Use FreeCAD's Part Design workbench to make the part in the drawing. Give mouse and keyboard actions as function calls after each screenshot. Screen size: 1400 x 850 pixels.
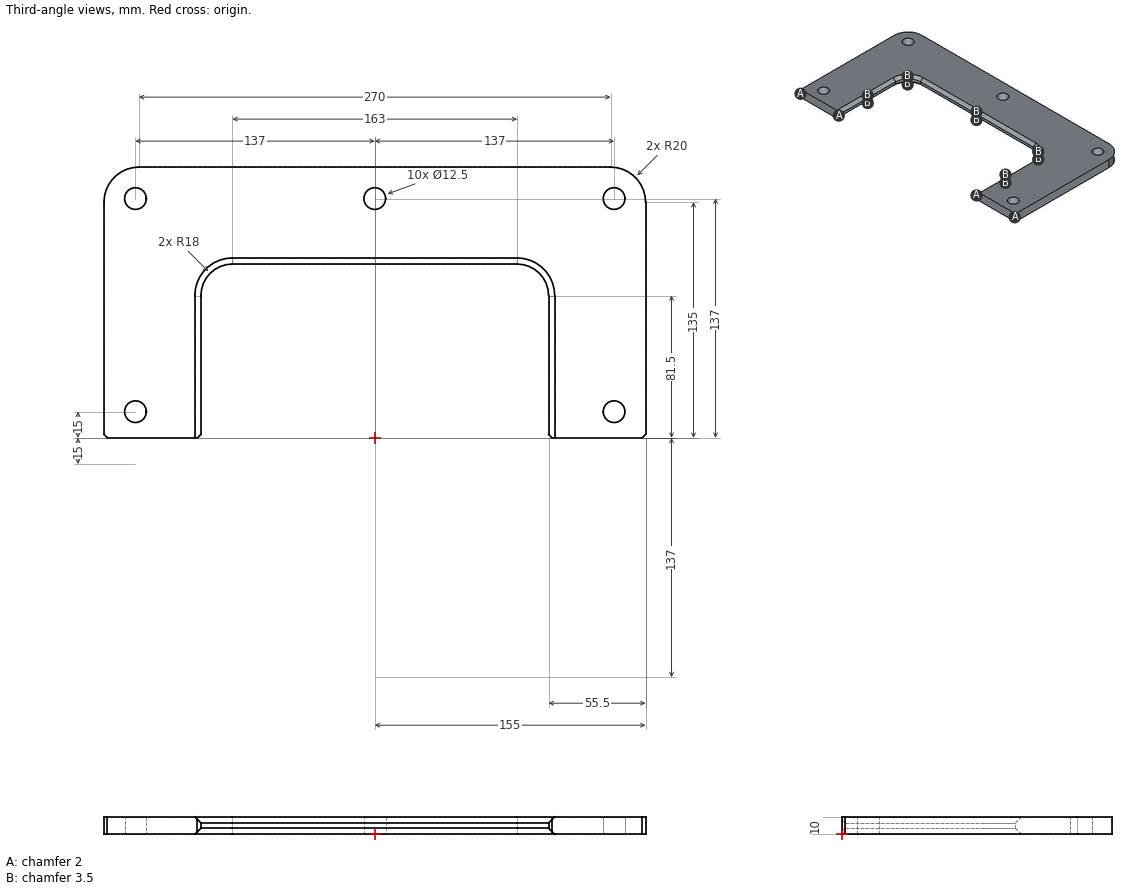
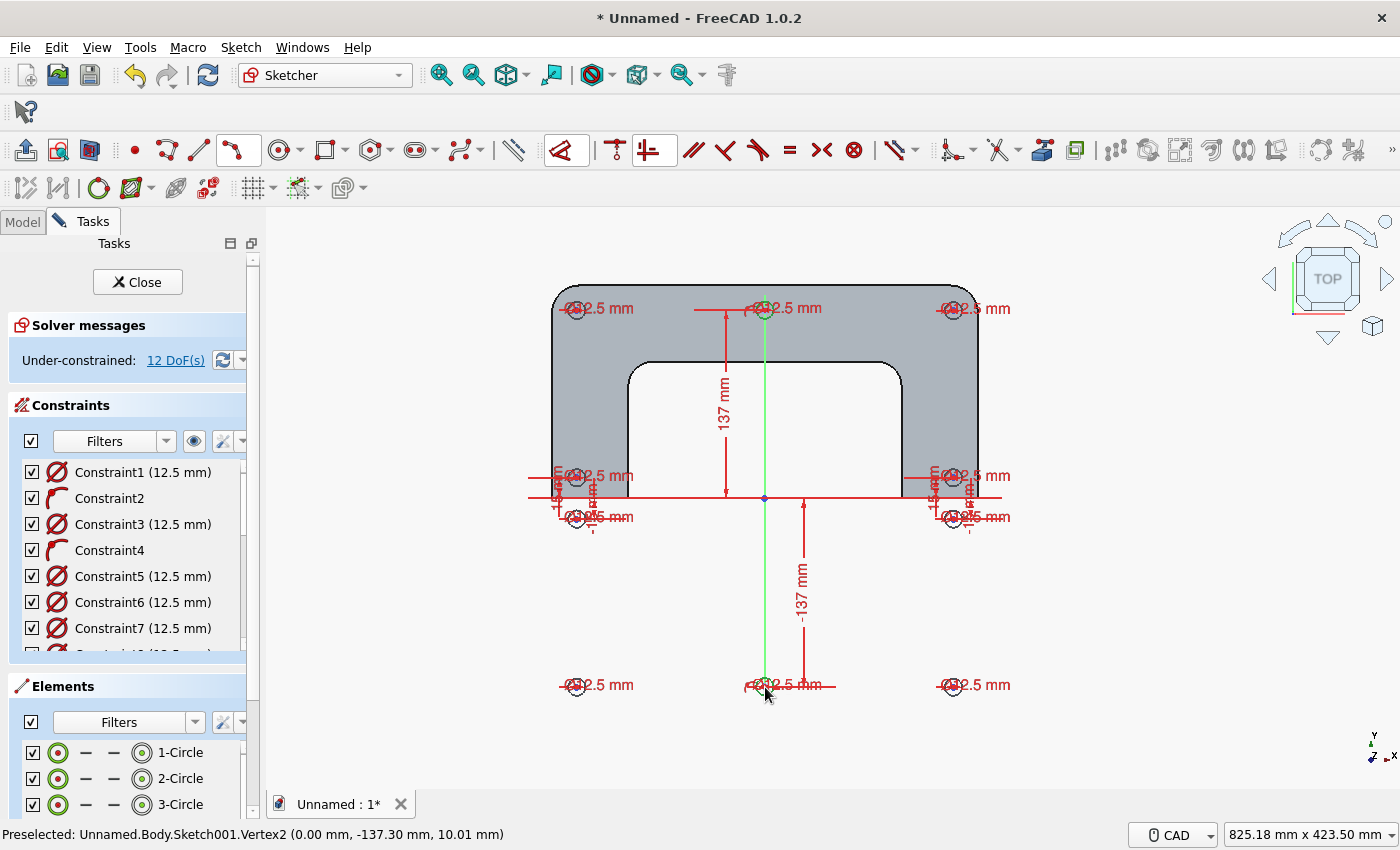
click(577, 310)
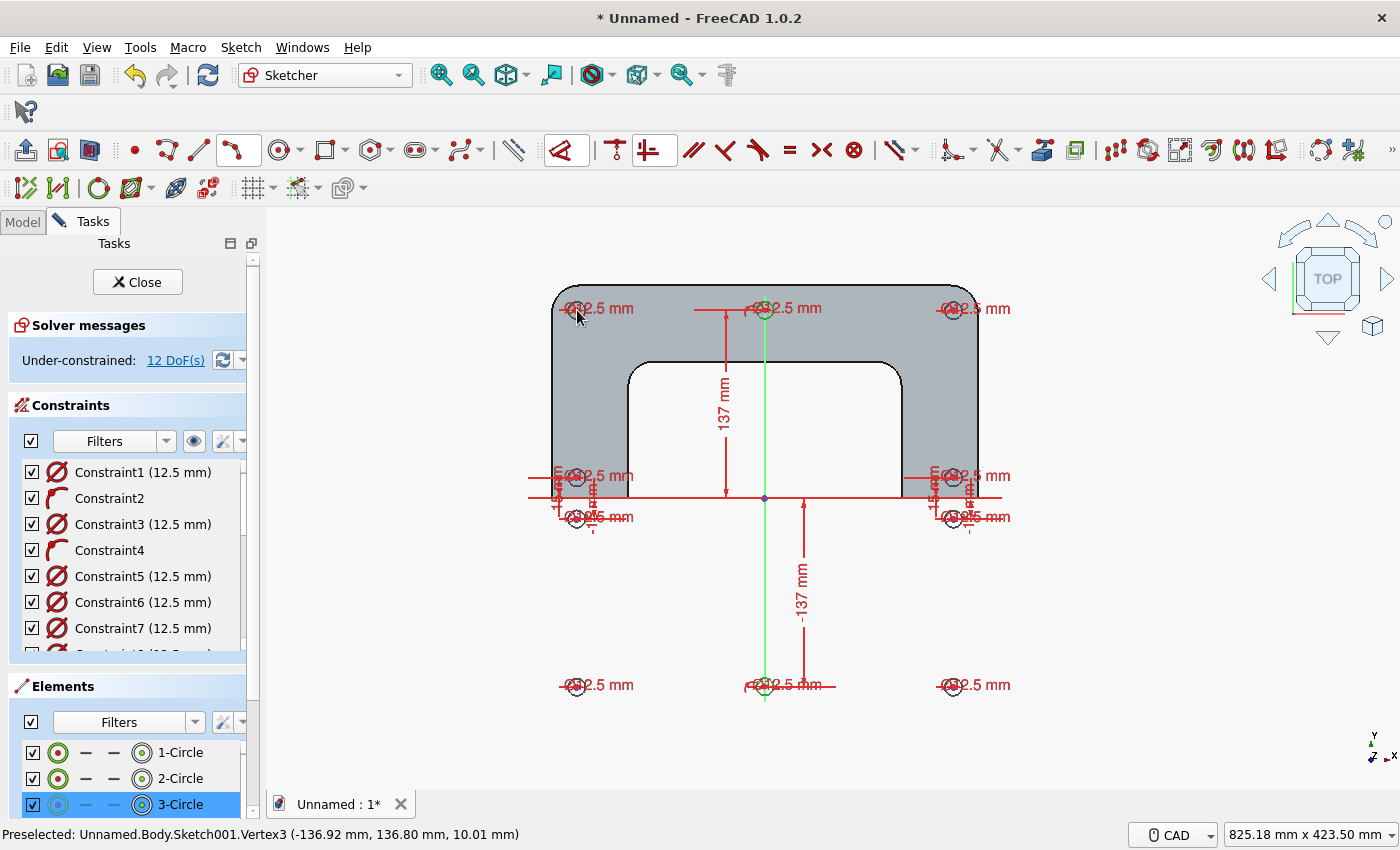
key(l)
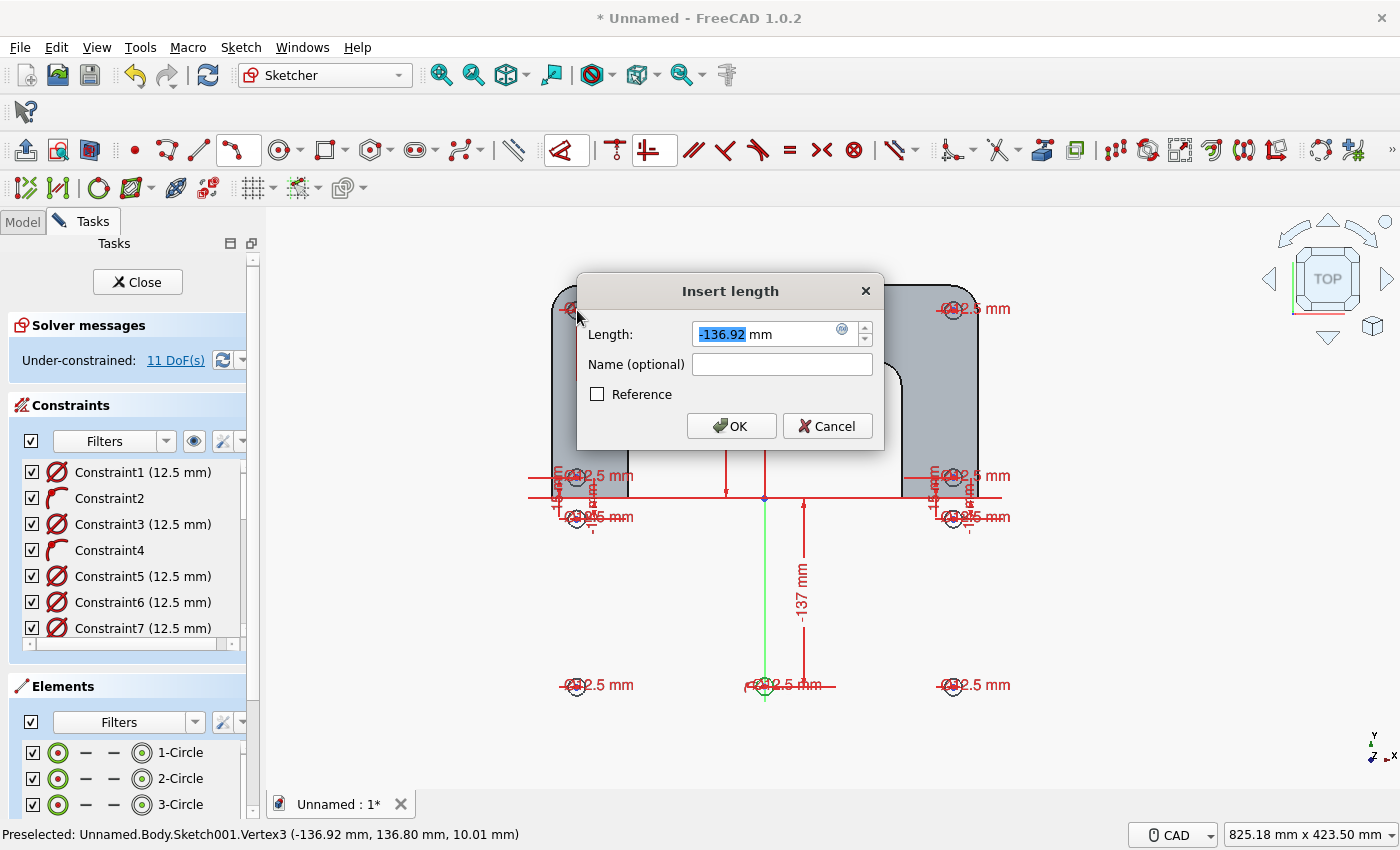
text(-137)
key(Return)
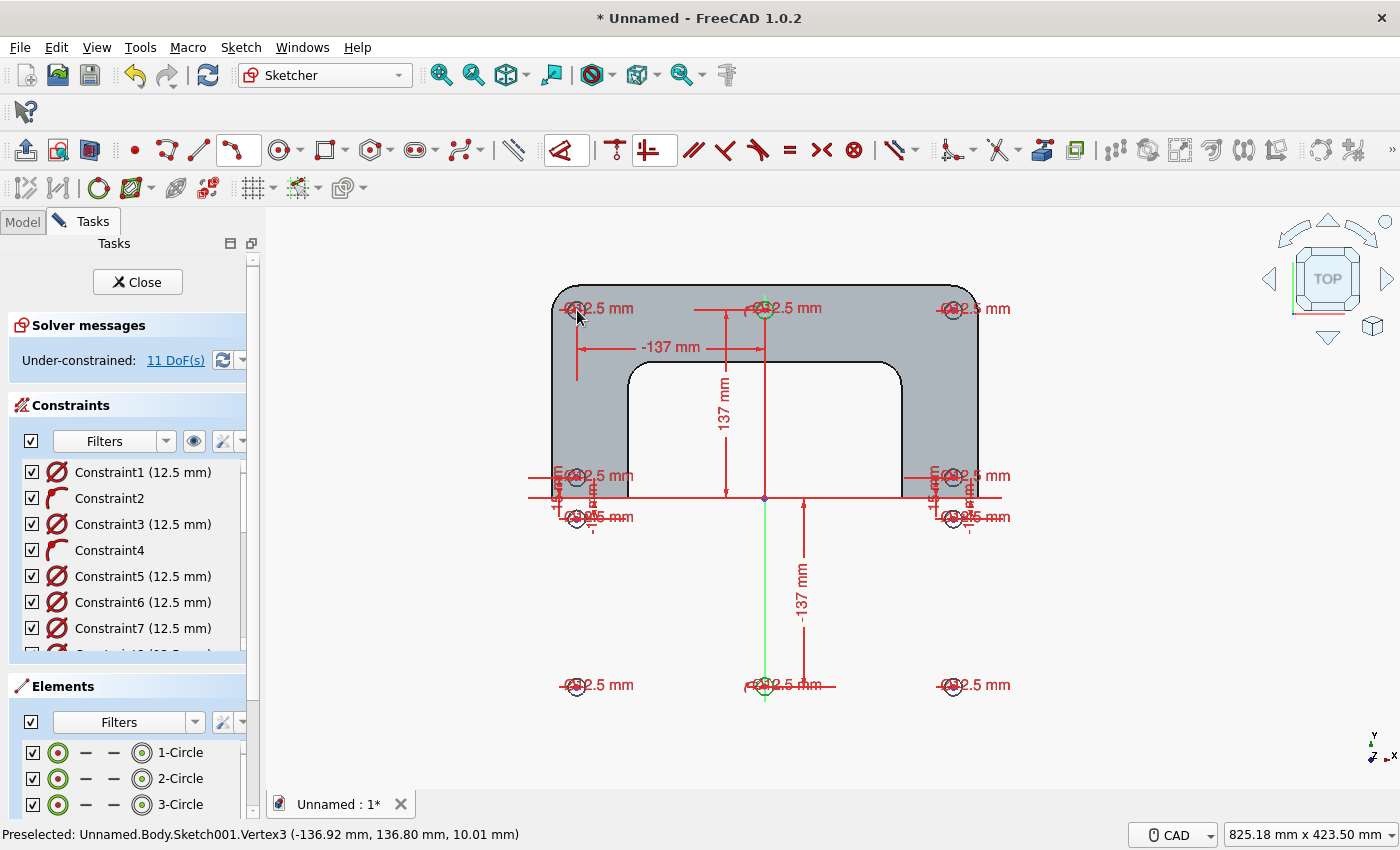
click(577, 310)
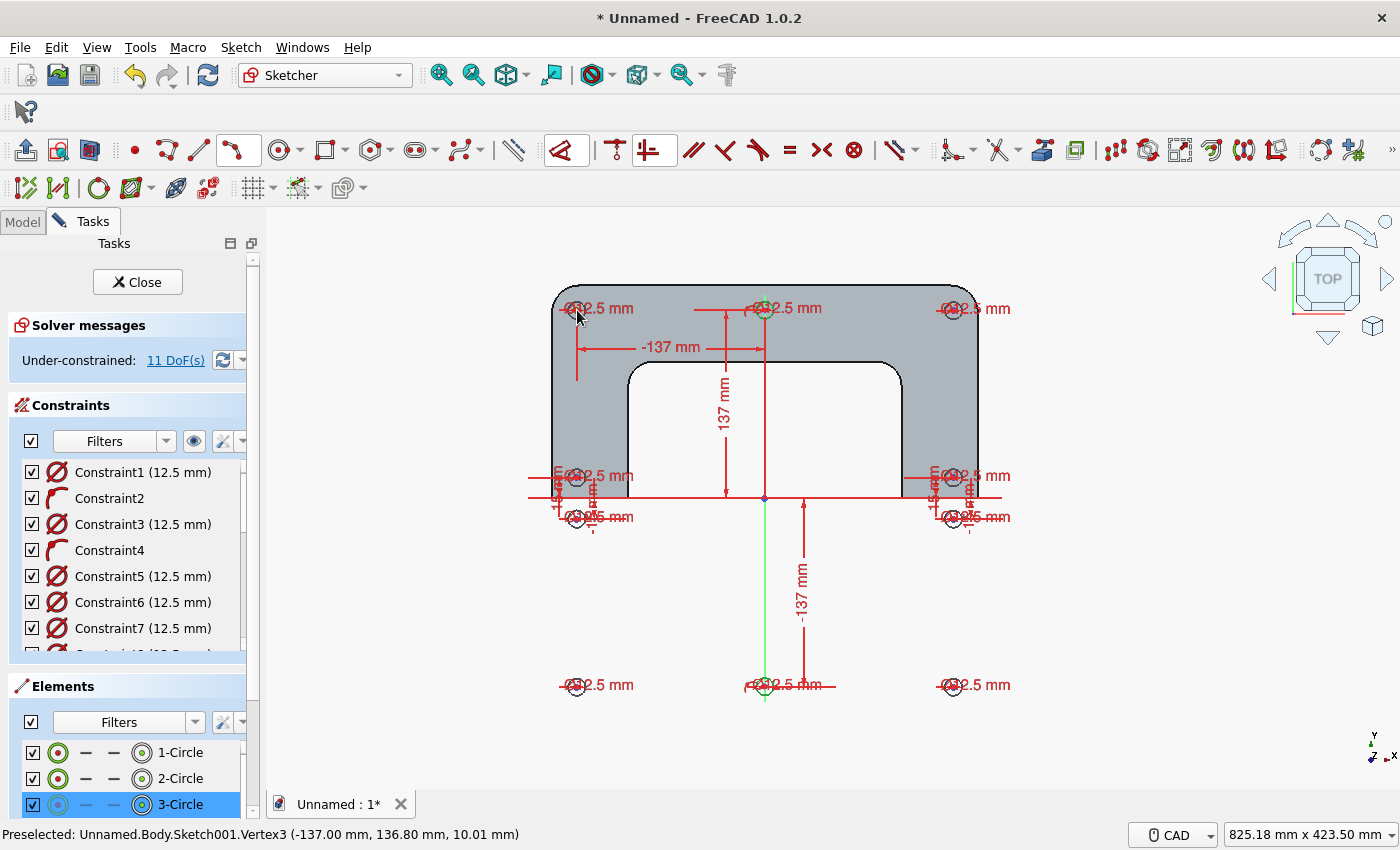
key(i)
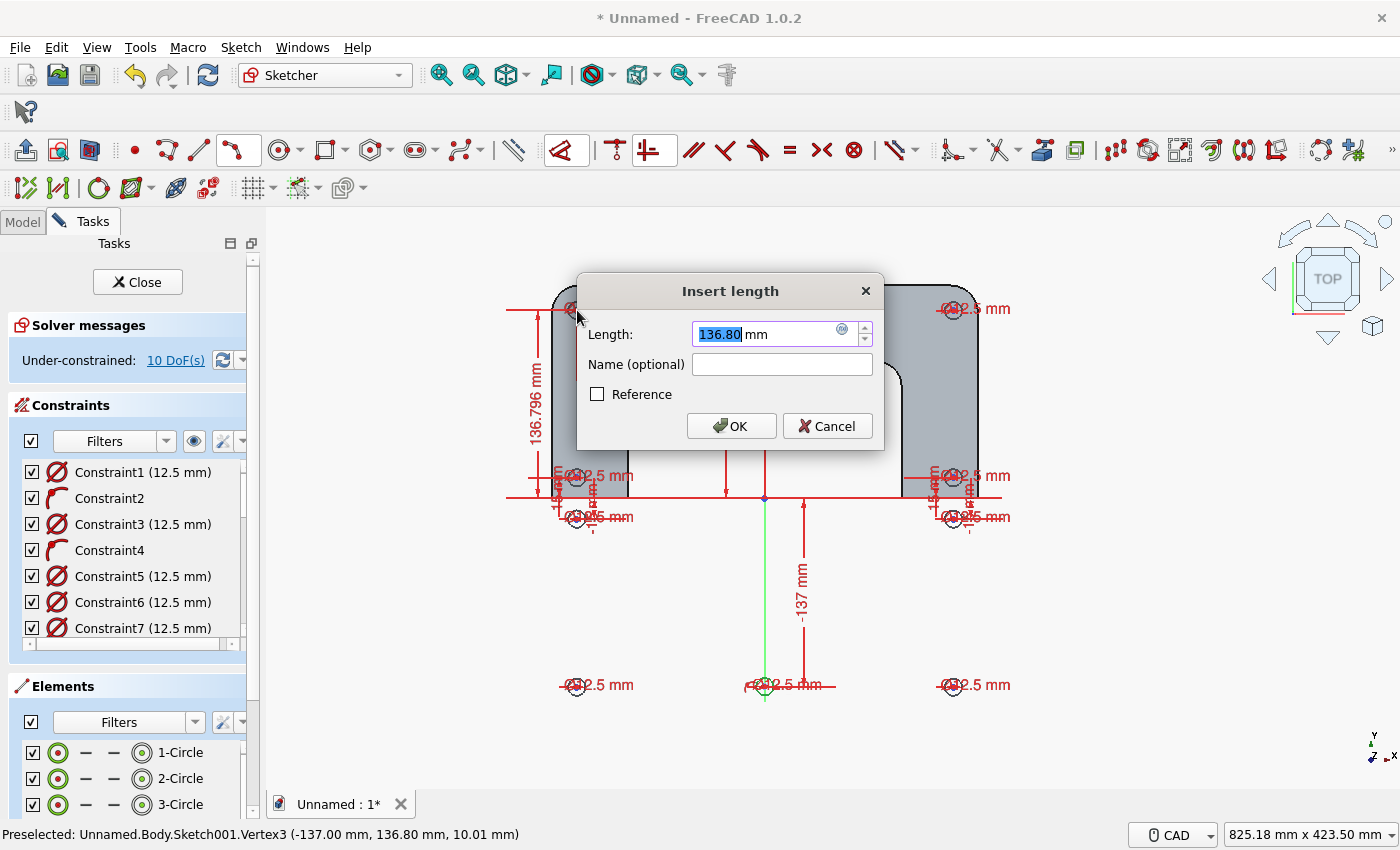
text(137)
key(Return)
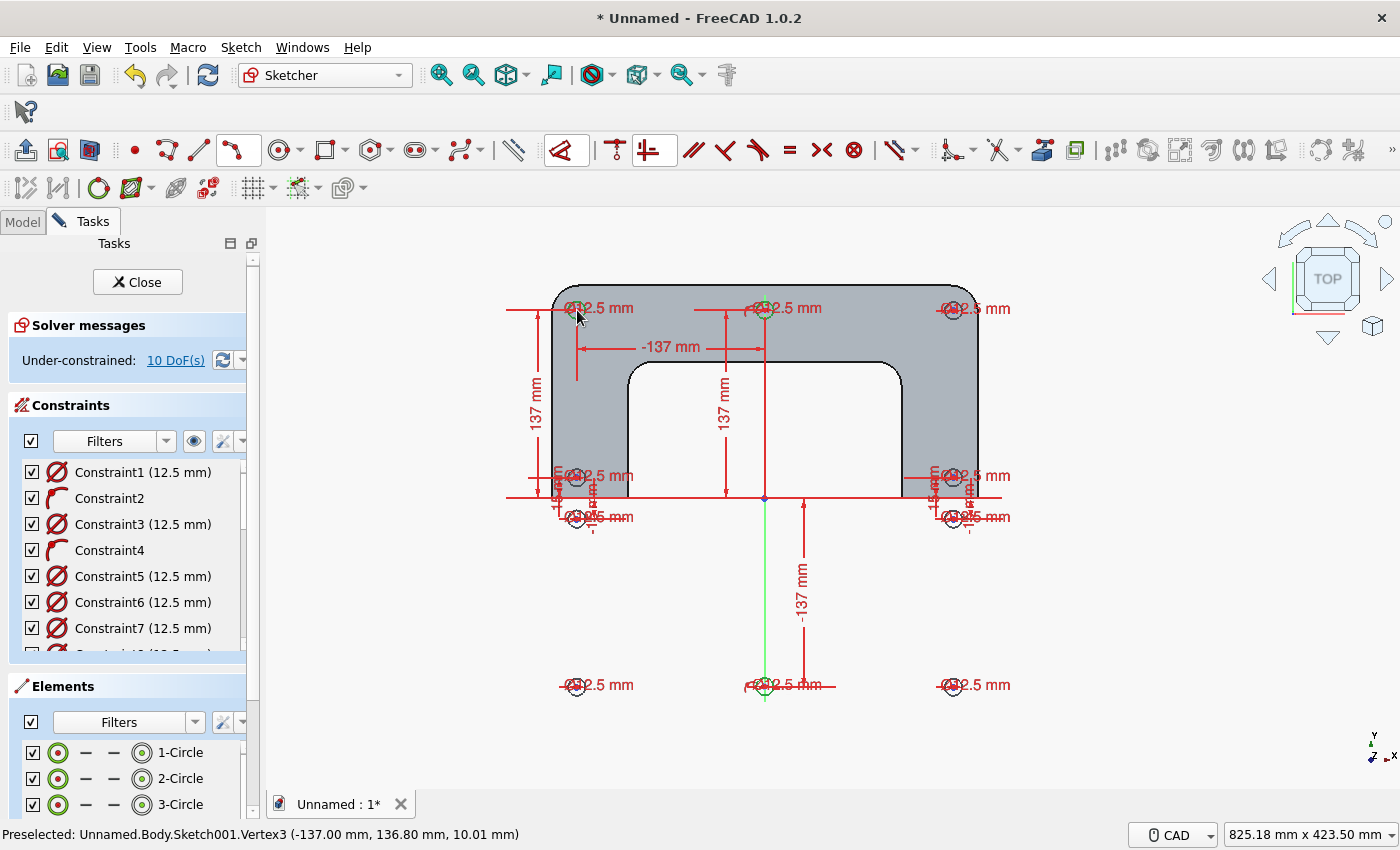
click(953, 311)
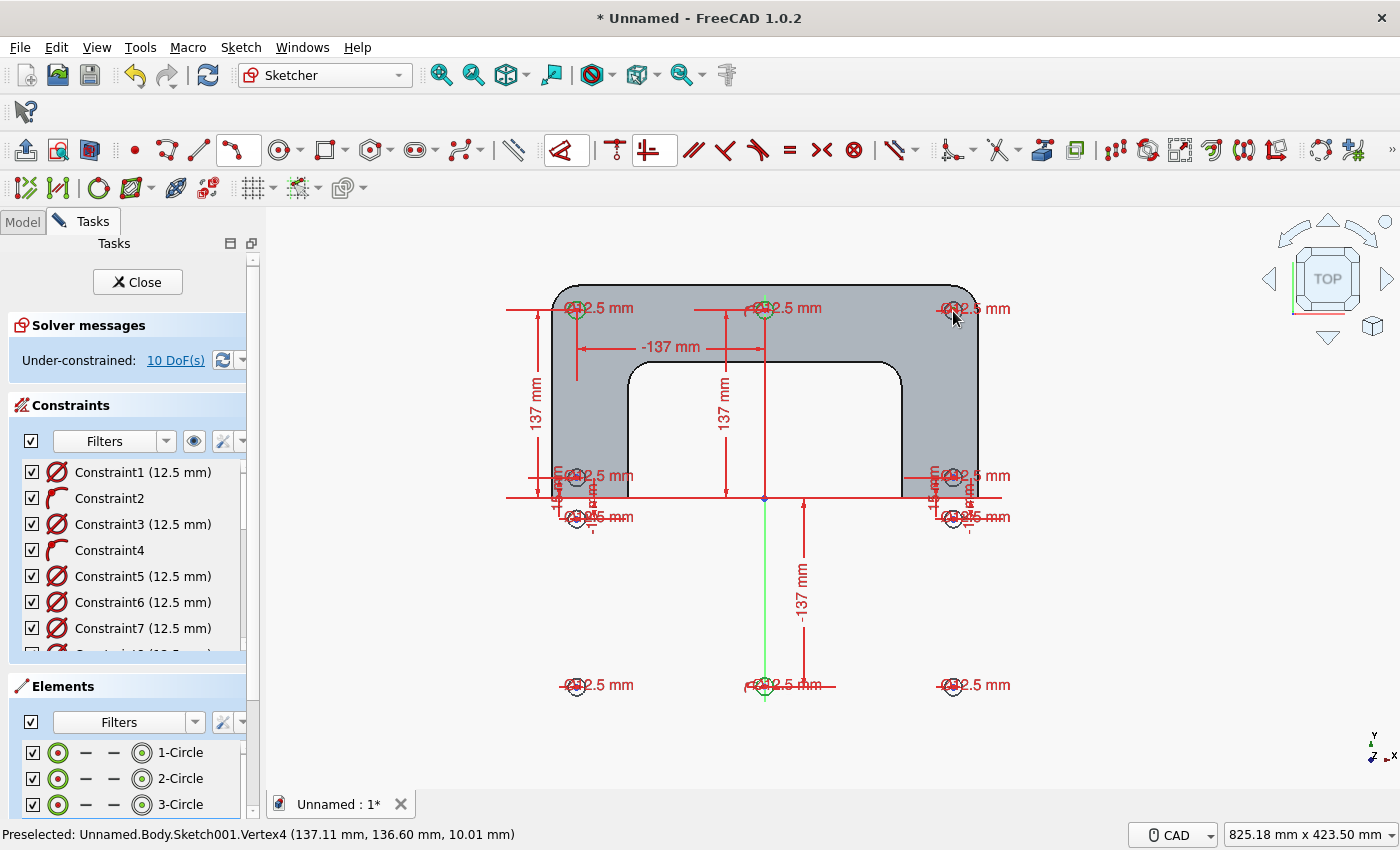
key(l)